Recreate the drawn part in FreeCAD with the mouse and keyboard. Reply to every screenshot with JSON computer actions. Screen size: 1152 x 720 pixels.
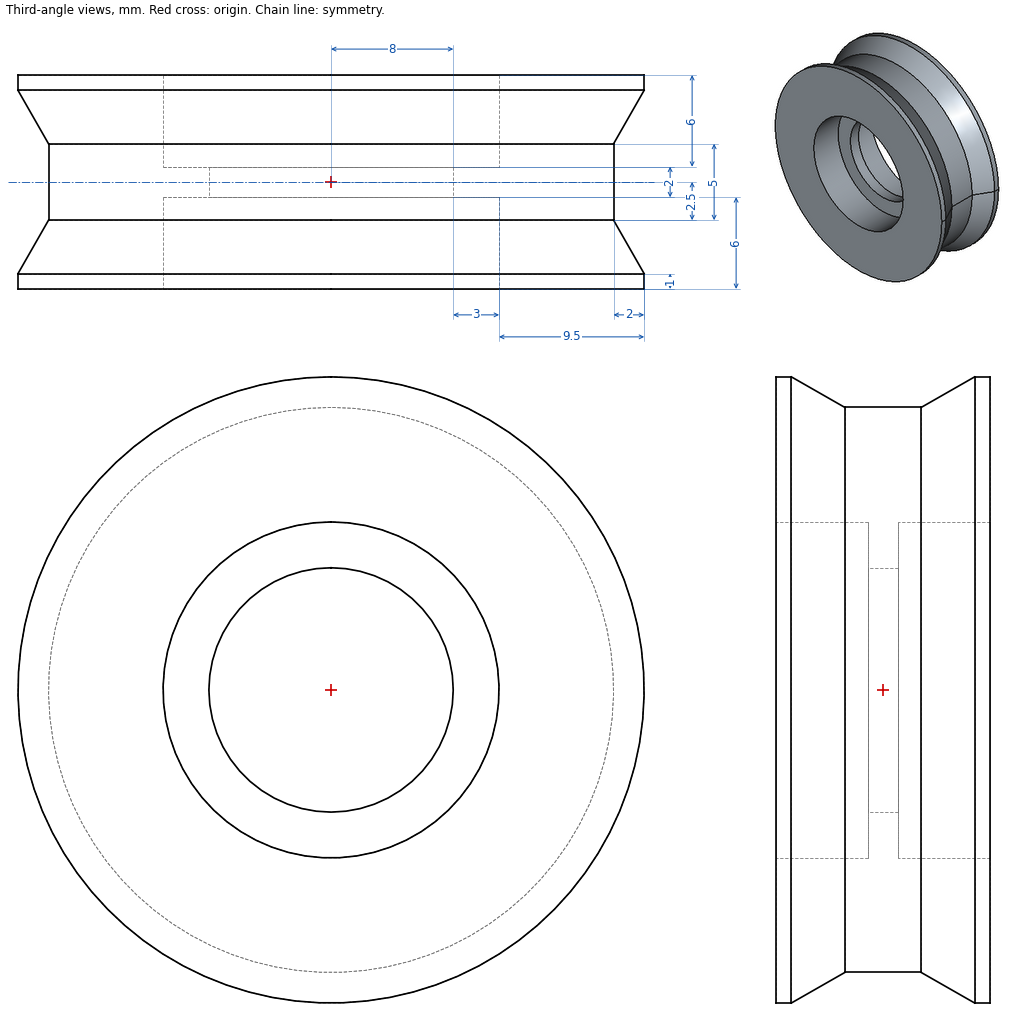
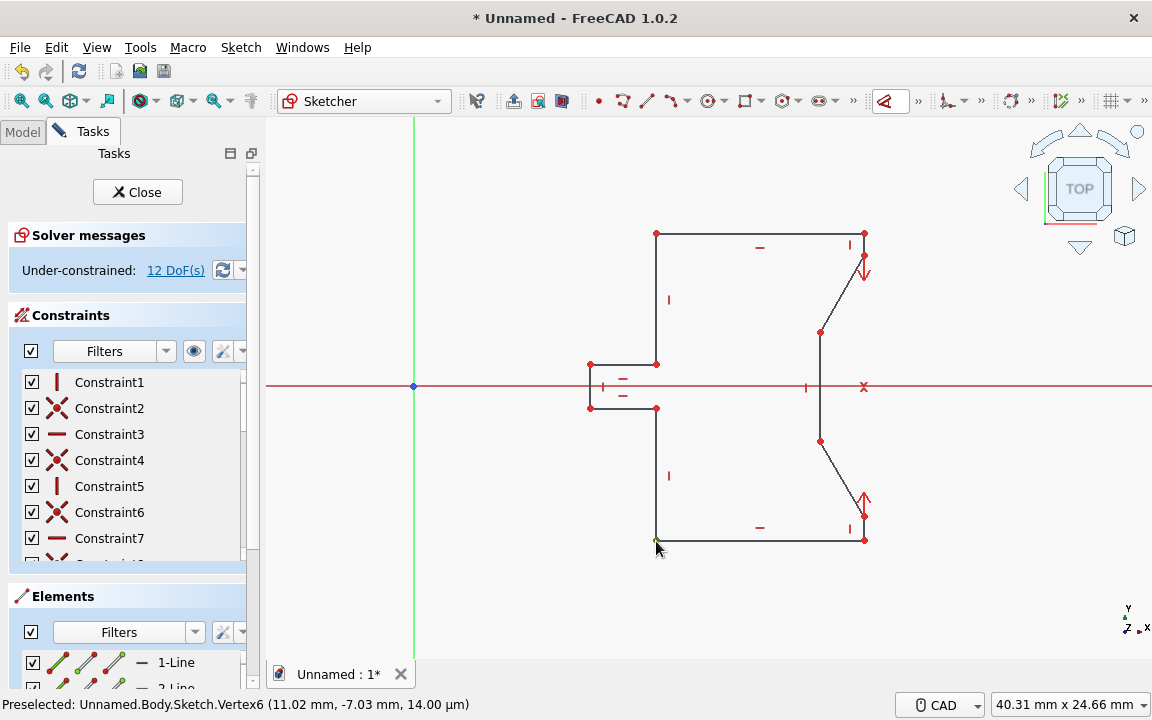
{"action": "left_click", "coordinate": [656, 234]}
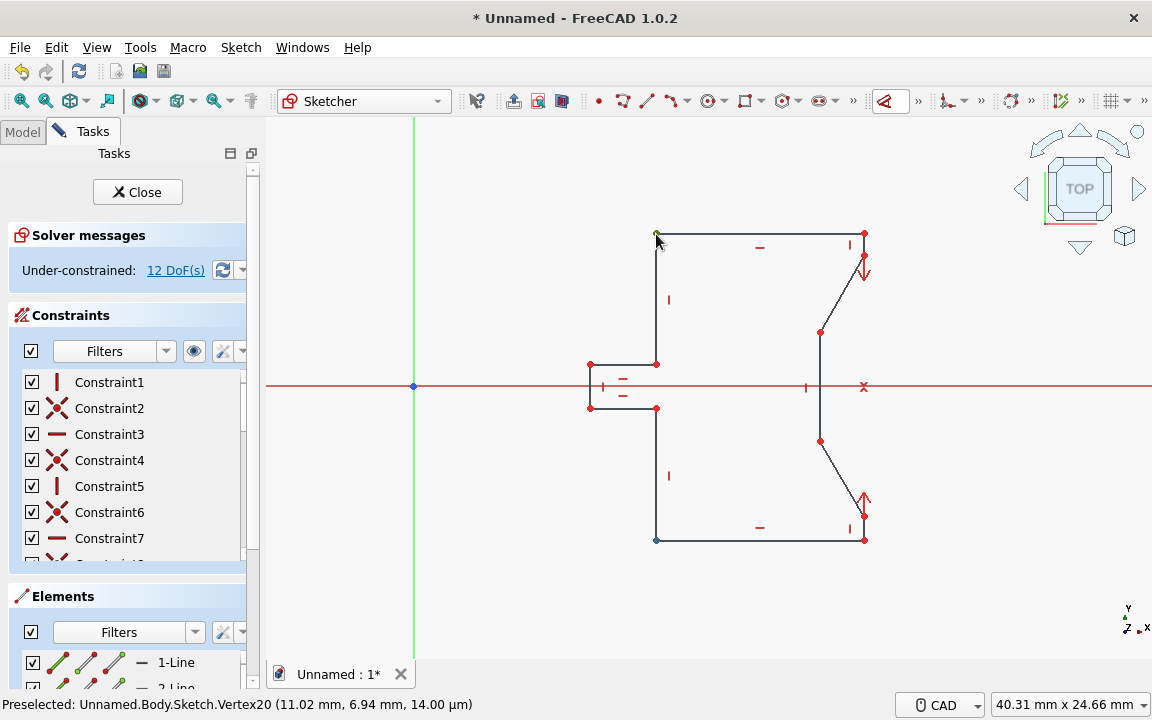
{"action": "left_click", "coordinate": [344, 386]}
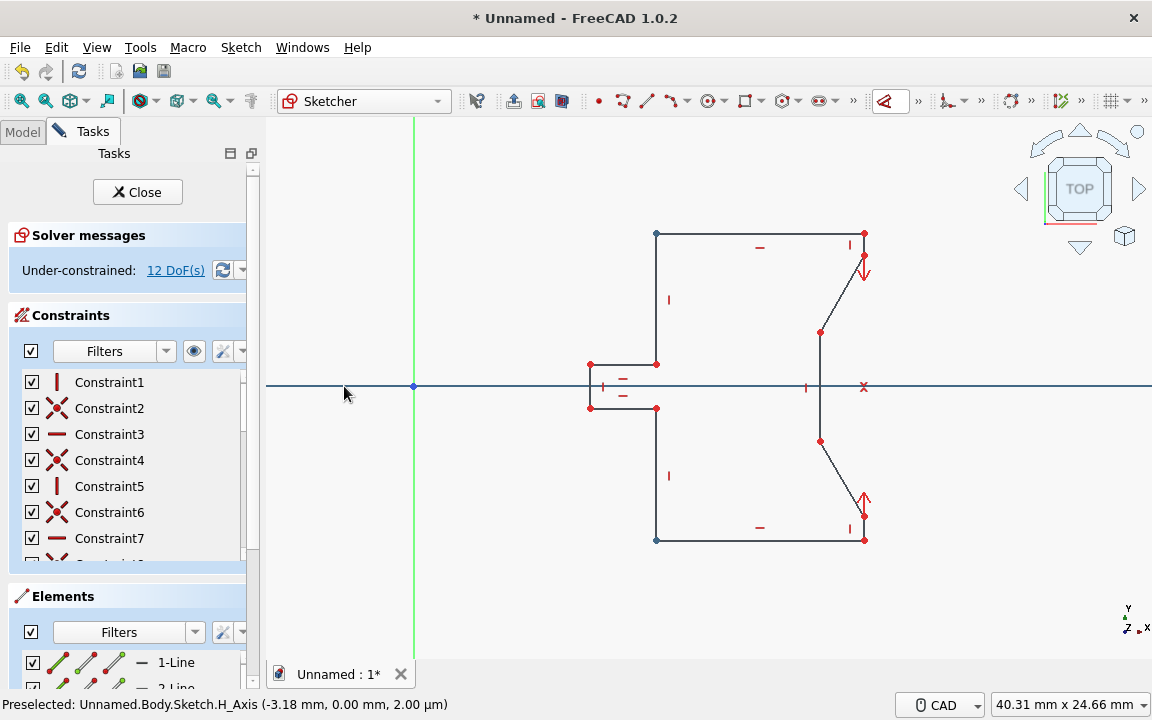
{"action": "key", "text": "s"}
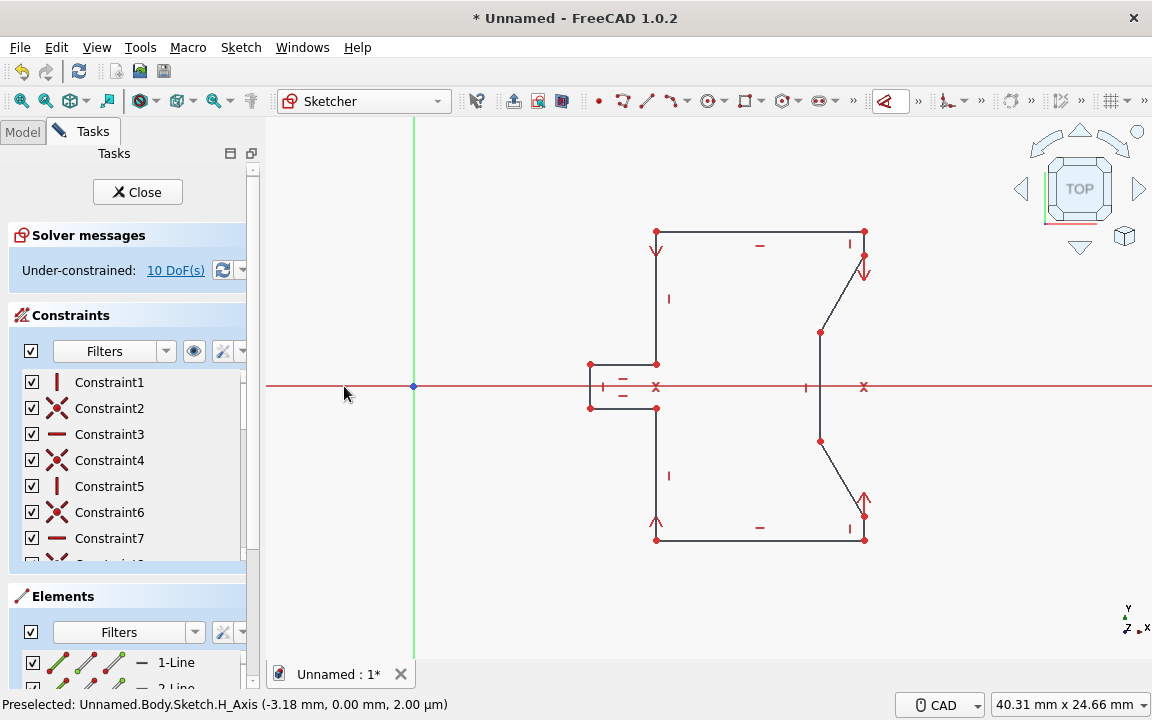
{"action": "left_click", "coordinate": [884, 102]}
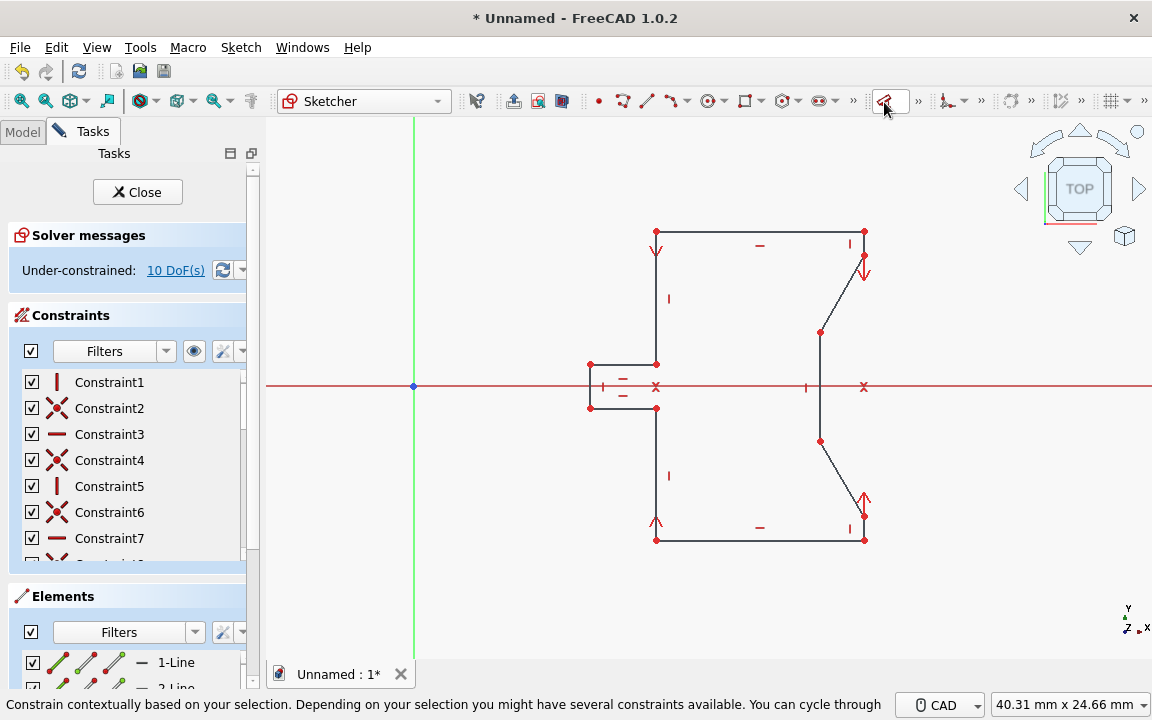
{"action": "scroll", "coordinate": [590, 396], "scroll_direction": "up", "scroll_amount": 2}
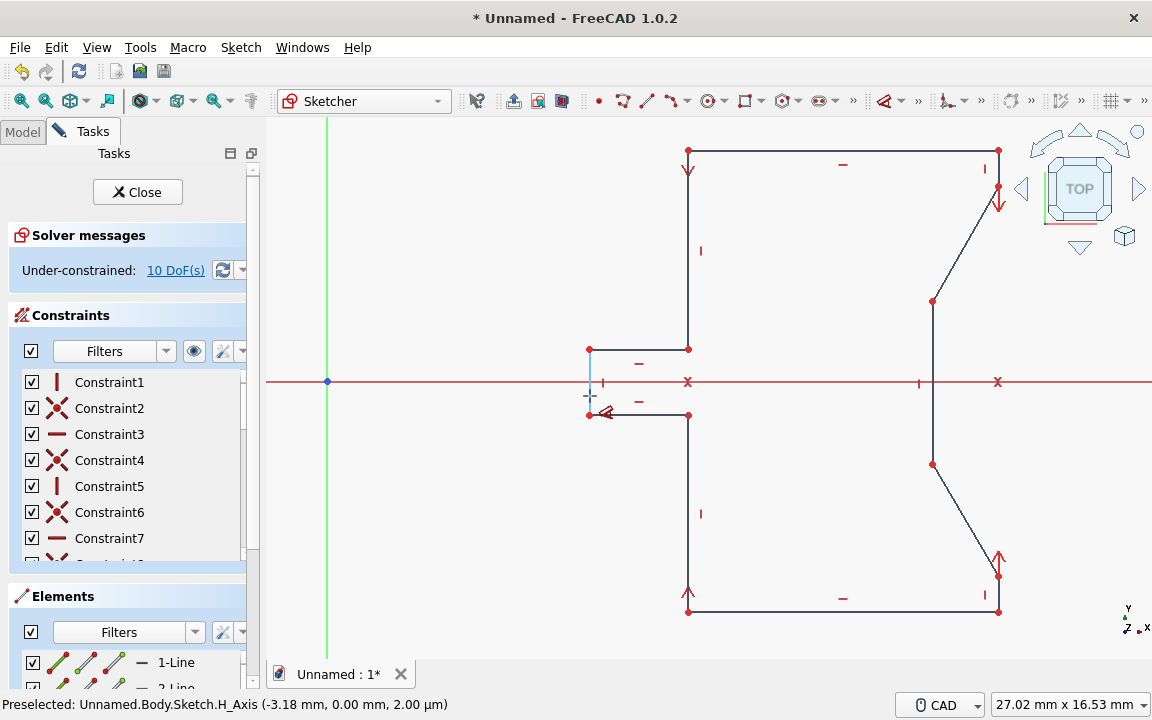
{"action": "left_click", "coordinate": [590, 395]}
{"action": "left_click", "coordinate": [556, 367]}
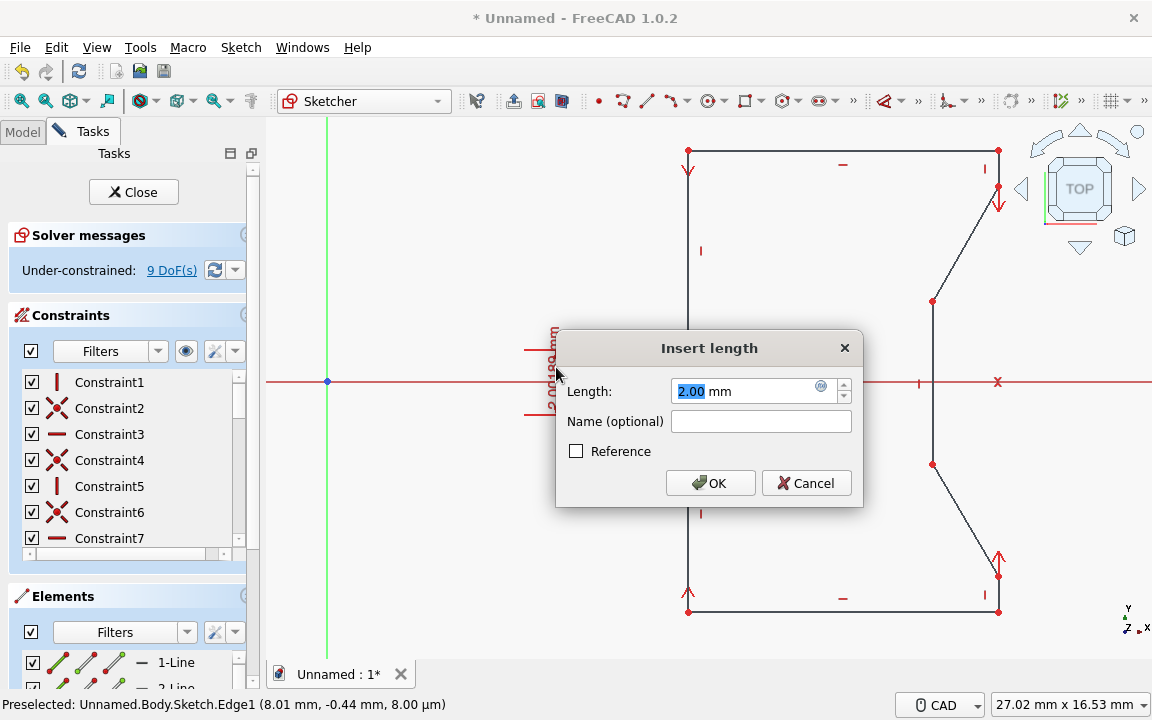
{"action": "type", "text": "2"}
{"action": "key", "text": "Return"}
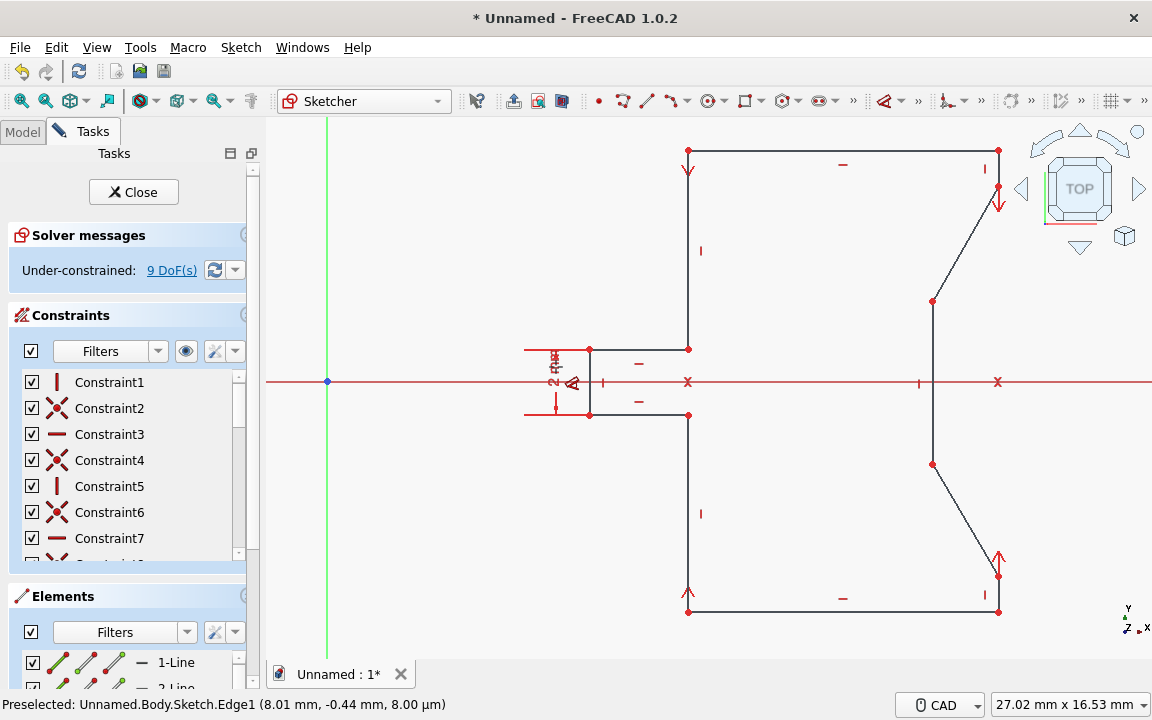
{"action": "left_click", "coordinate": [619, 415]}
{"action": "left_click", "coordinate": [639, 449]}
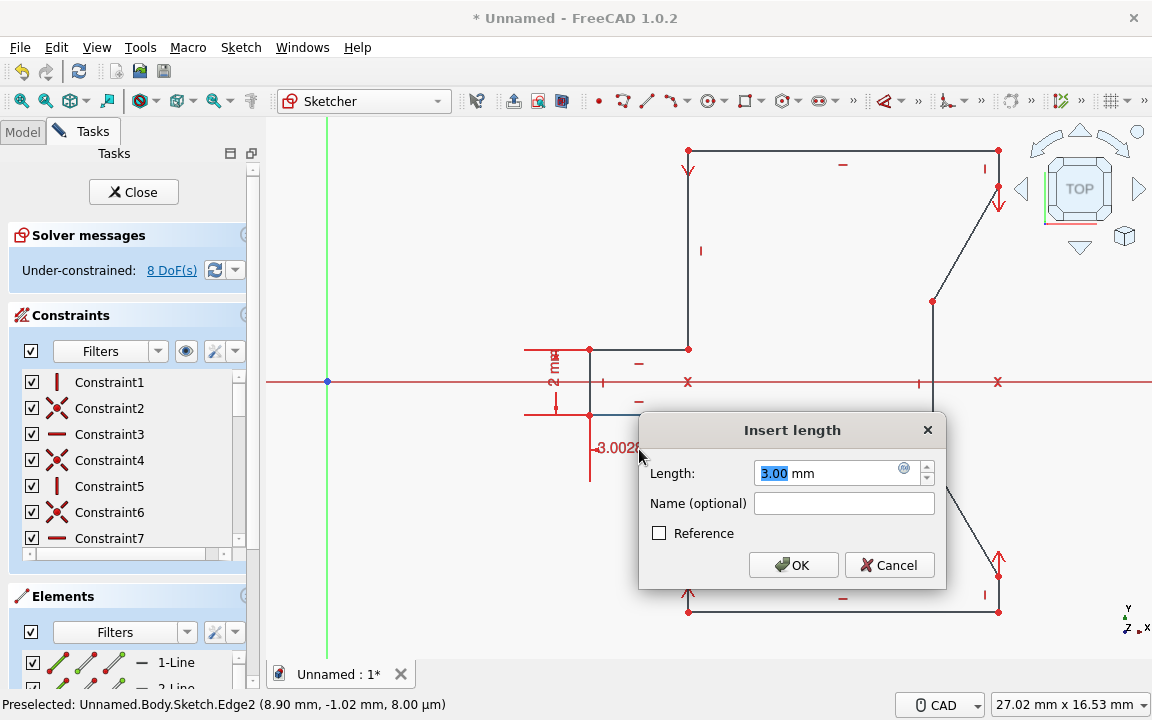
{"action": "type", "text": "3"}
{"action": "key", "text": "Return"}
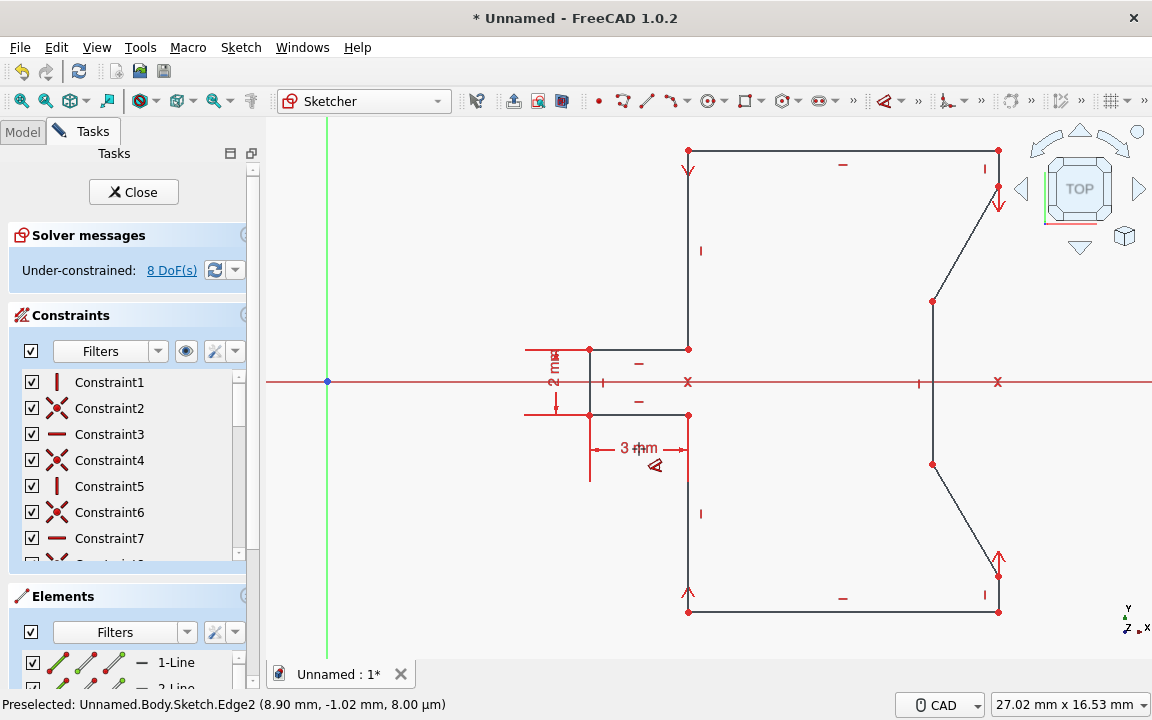
{"action": "left_click", "coordinate": [688, 474]}
{"action": "left_click", "coordinate": [722, 514]}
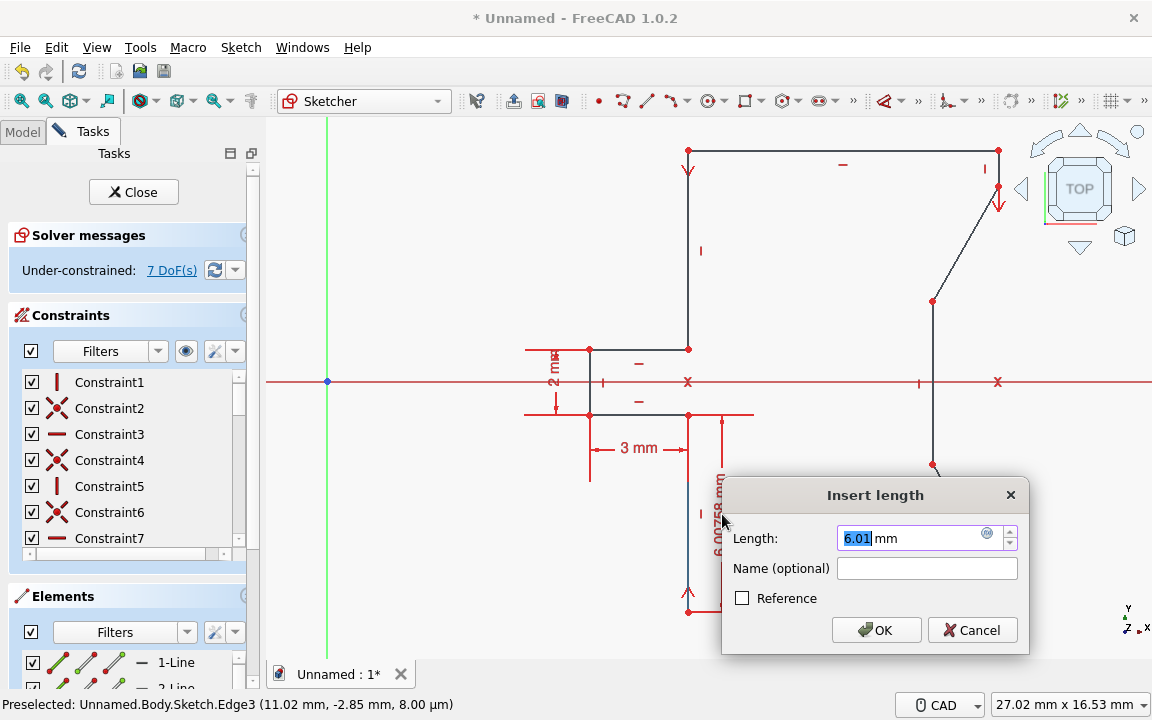
{"action": "type", "text": "6"}
{"action": "key", "text": "Return"}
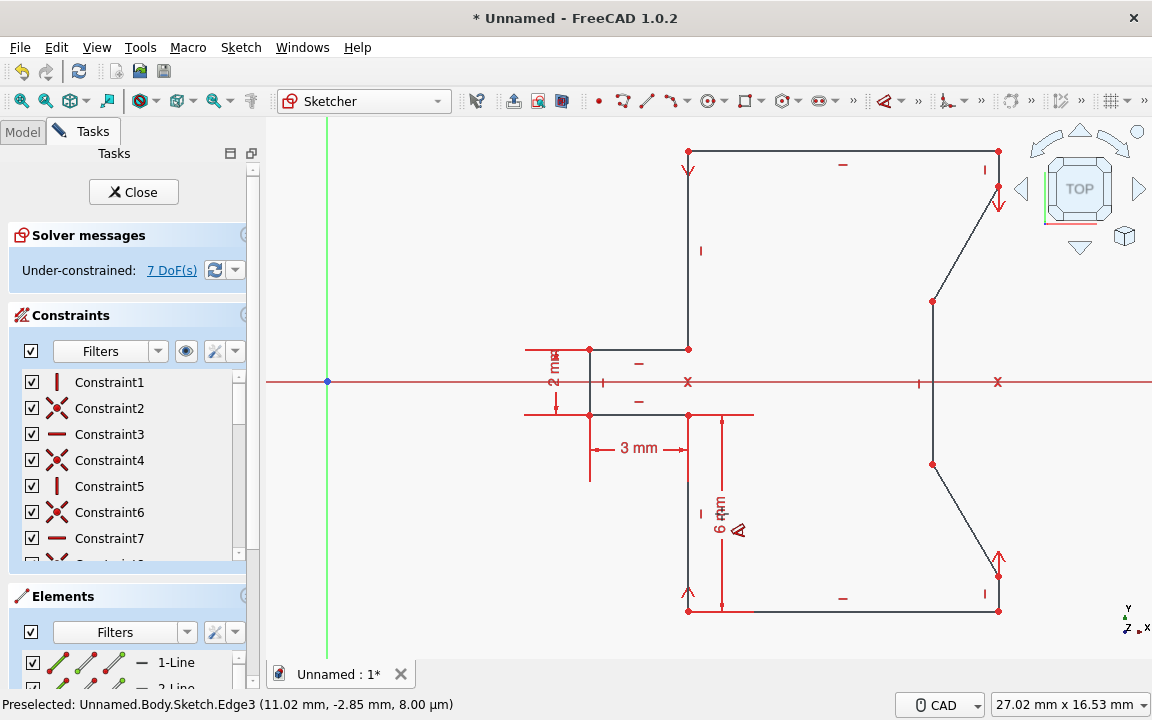
{"action": "scroll", "coordinate": [595, 401], "scroll_direction": "down", "scroll_amount": 2}